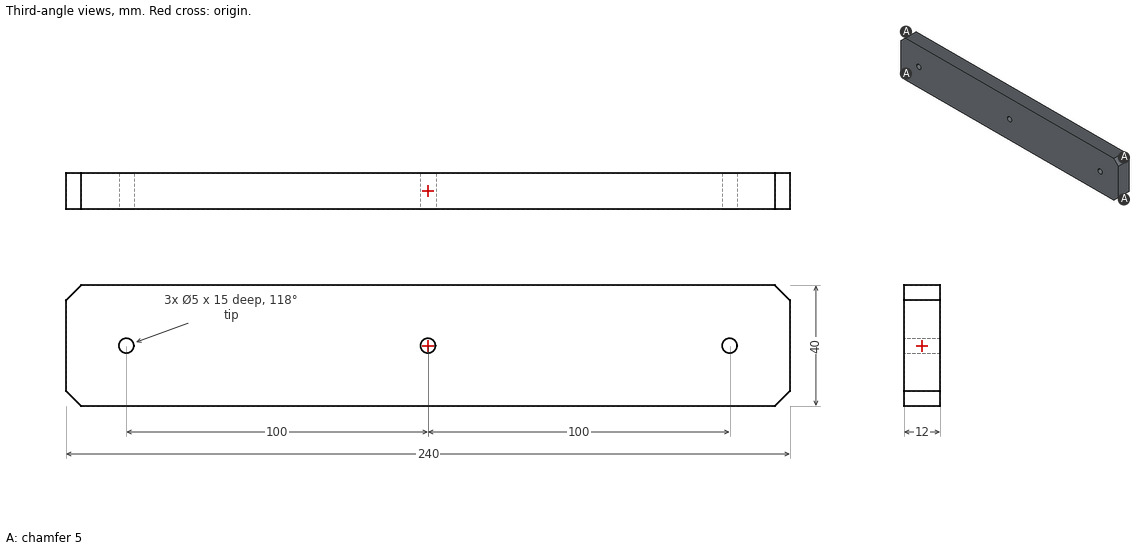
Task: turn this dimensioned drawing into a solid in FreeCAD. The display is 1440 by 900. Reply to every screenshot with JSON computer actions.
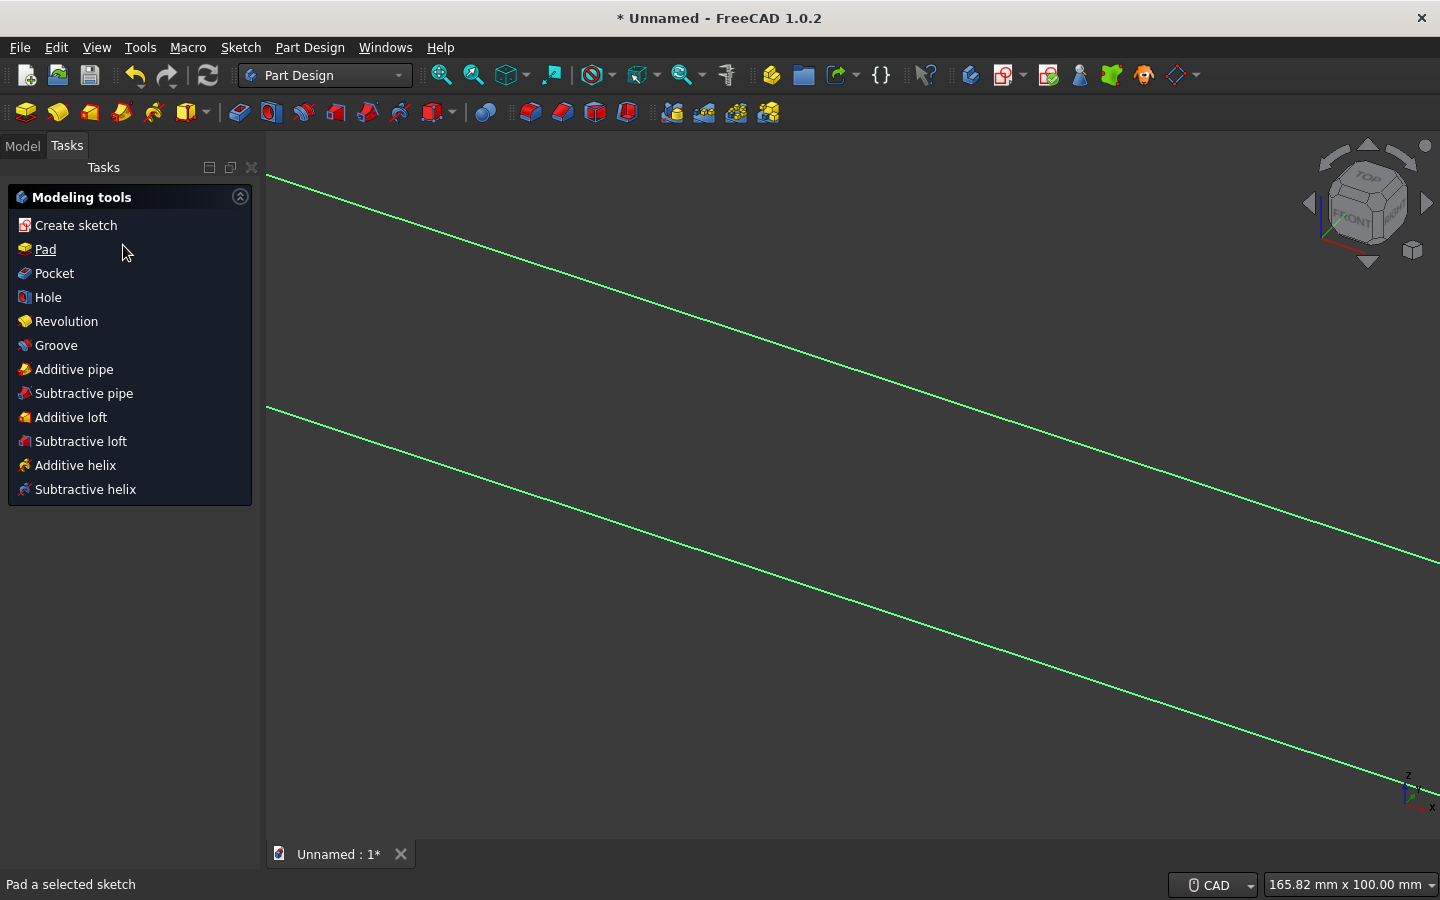
{"action": "left_click", "coordinate": [26, 112]}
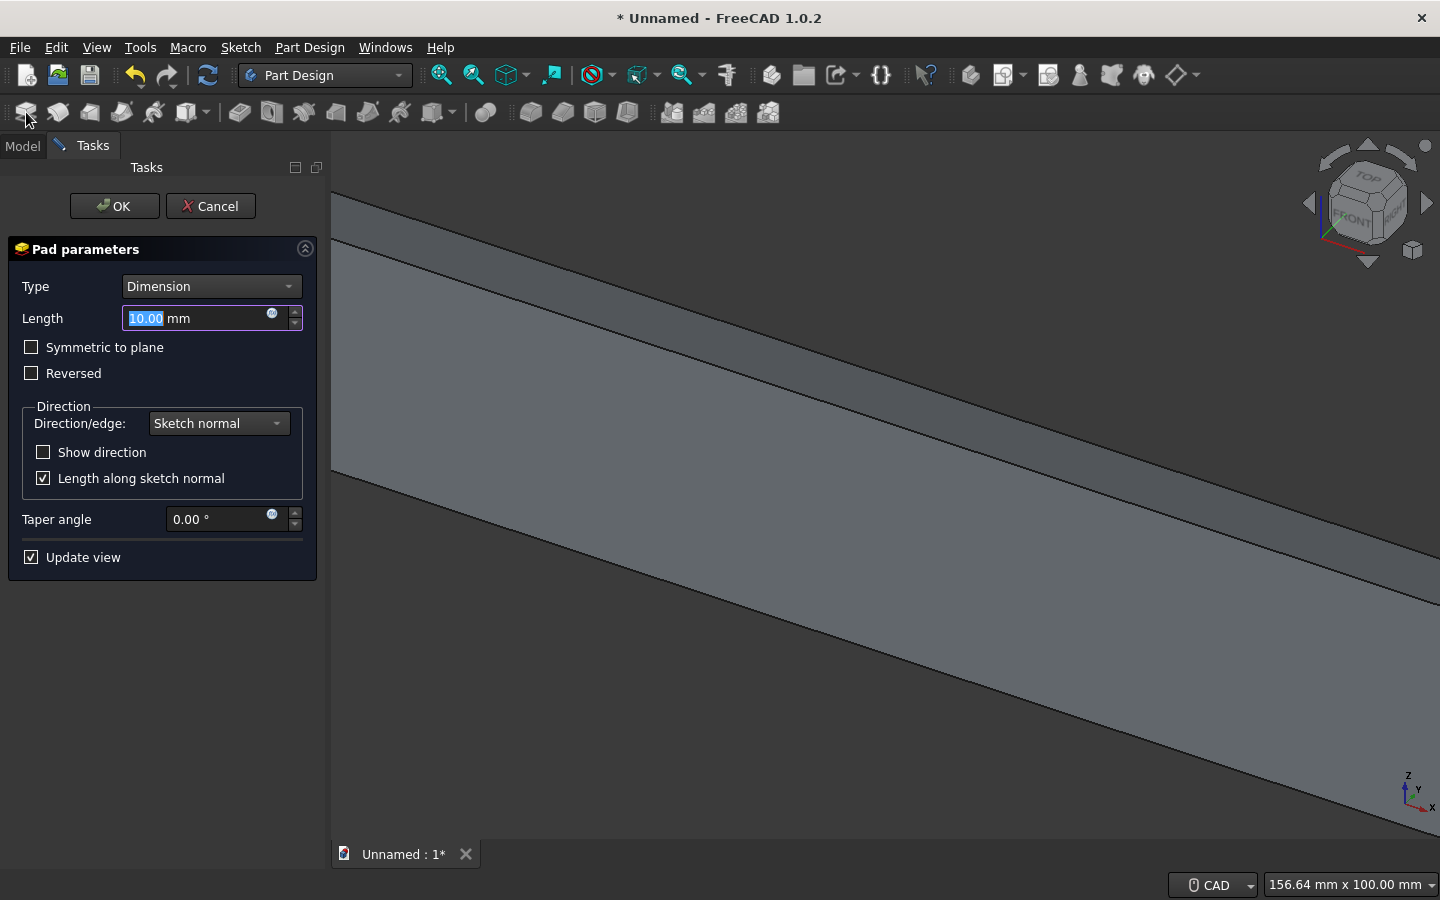
{"action": "type", "text": "12"}
{"action": "key", "text": "Tab"}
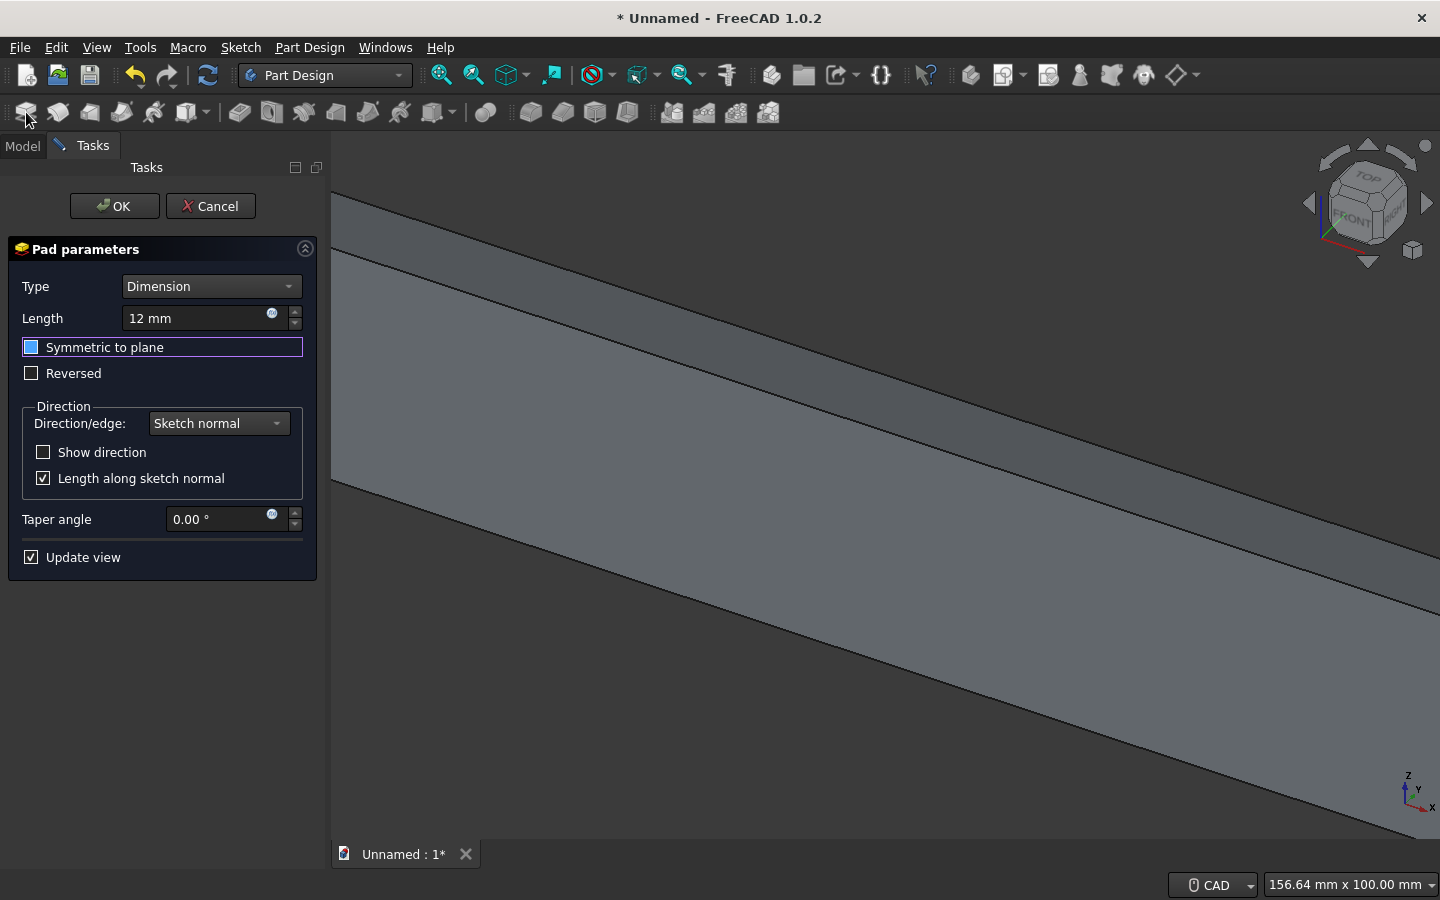
{"action": "left_click", "coordinate": [30, 347]}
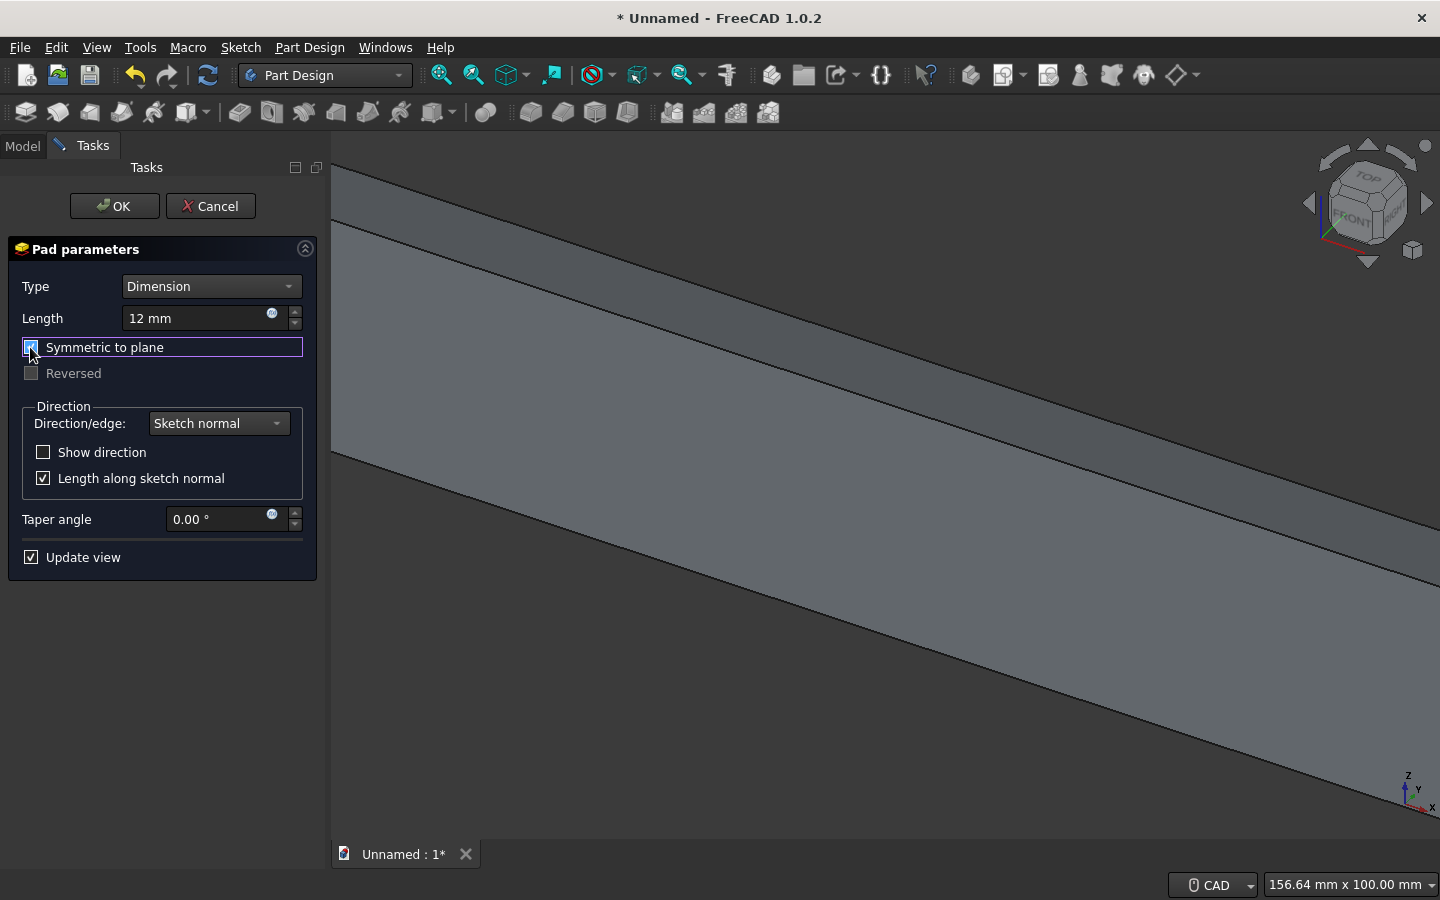
{"action": "left_click", "coordinate": [115, 206]}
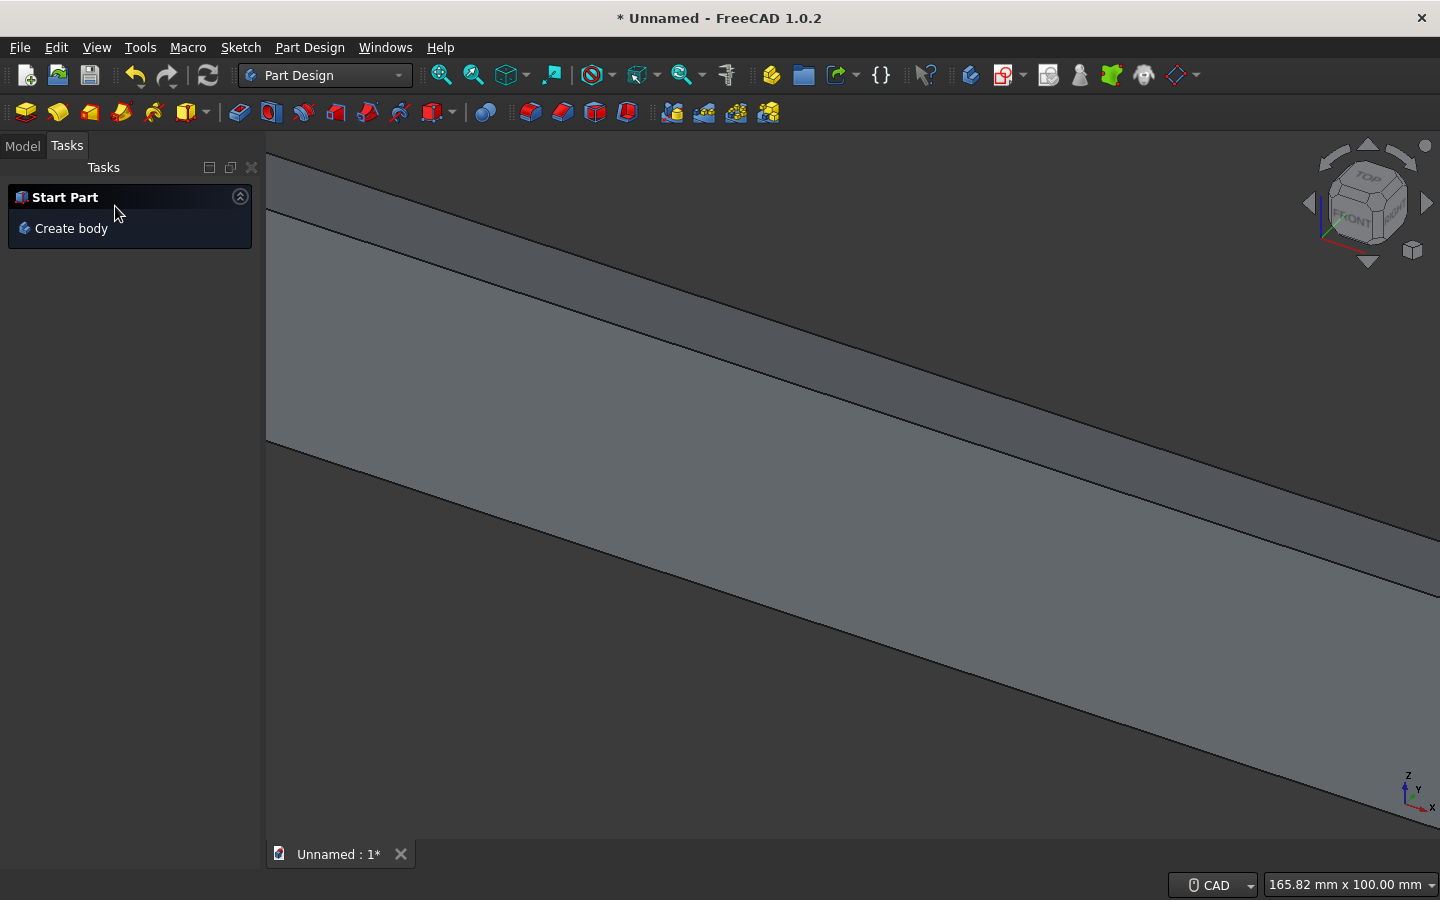
{"action": "left_click", "coordinate": [442, 76]}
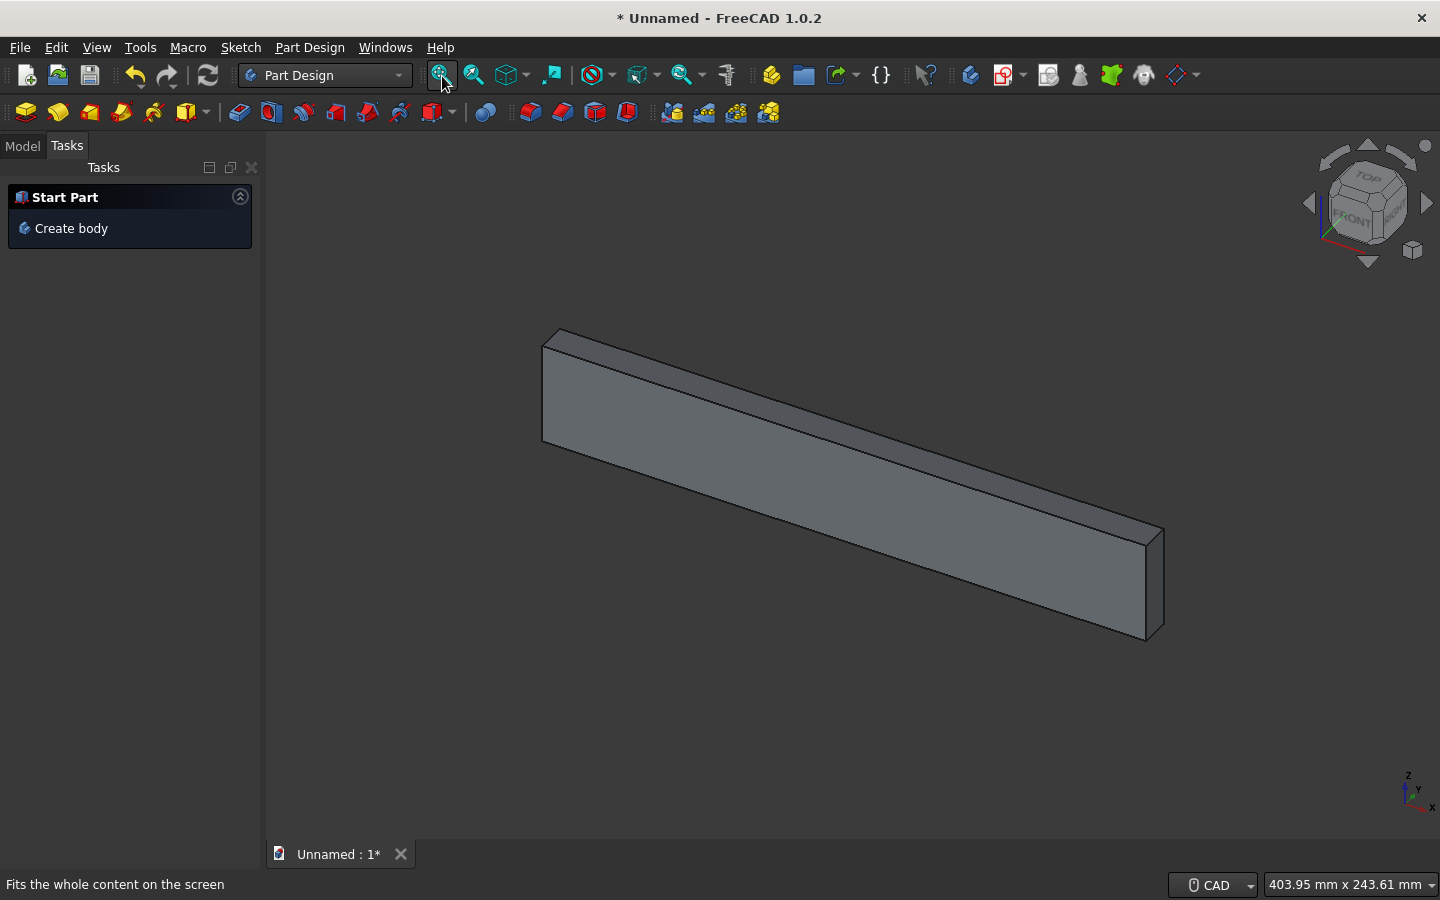
{"action": "key", "text": "4"}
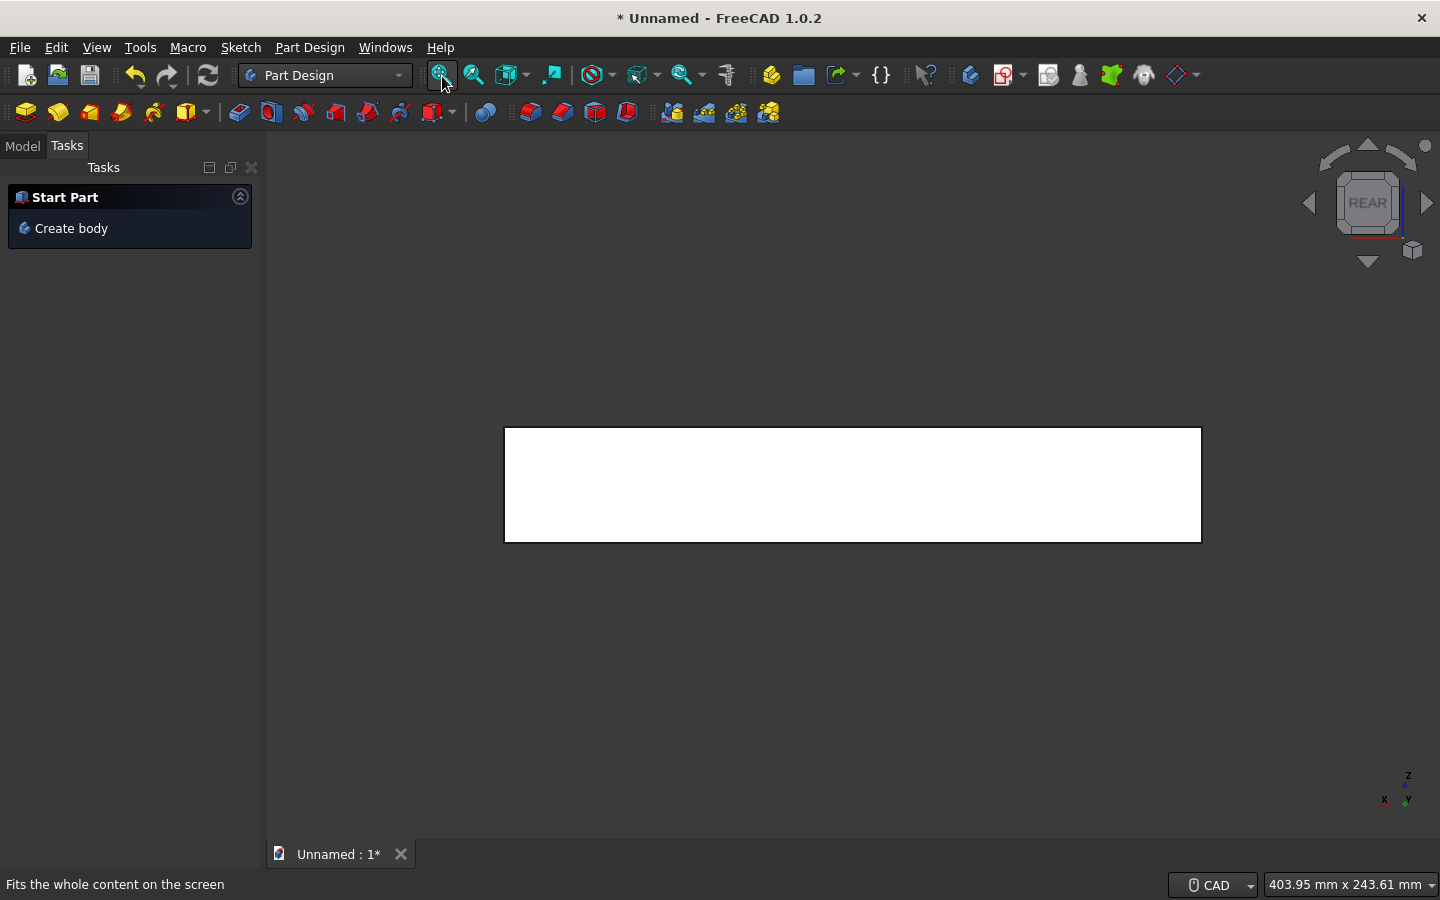
{"action": "left_click", "coordinate": [654, 484]}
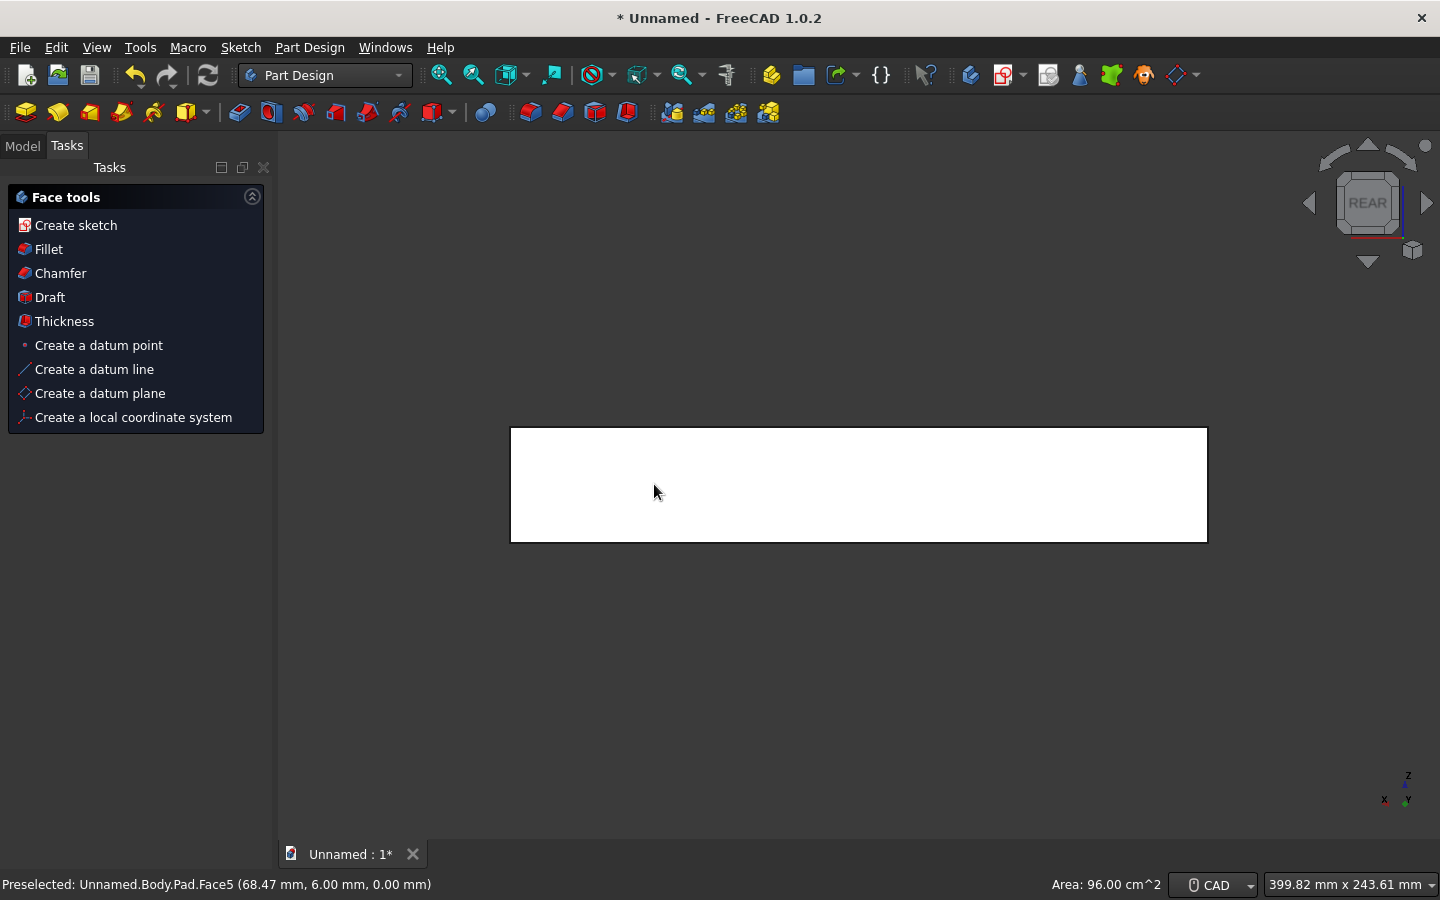
{"action": "left_click", "coordinate": [1004, 76]}